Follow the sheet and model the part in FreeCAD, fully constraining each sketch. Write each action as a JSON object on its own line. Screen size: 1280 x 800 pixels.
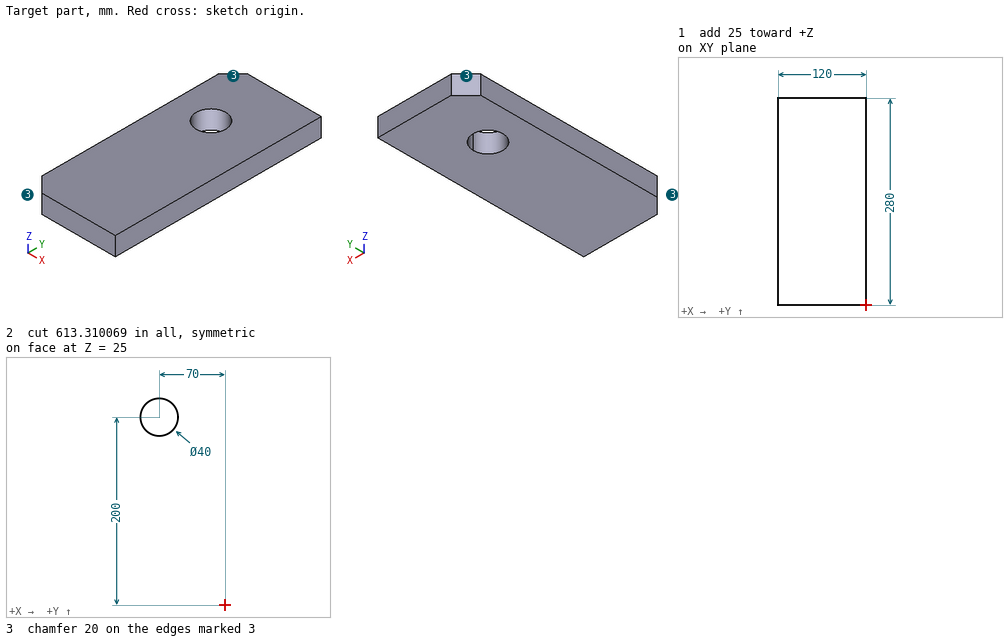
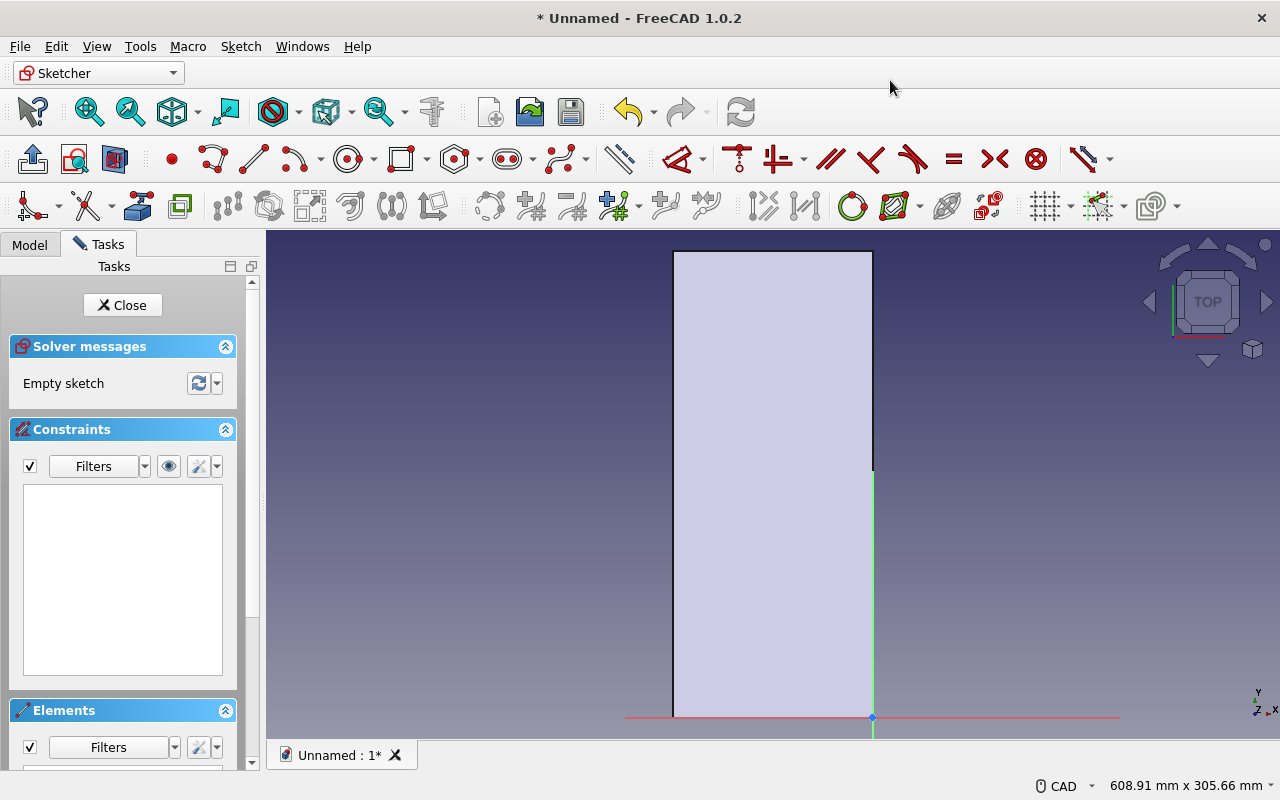
{"action": "scroll", "coordinate": [769, 359], "scroll_direction": "up", "scroll_amount": 8}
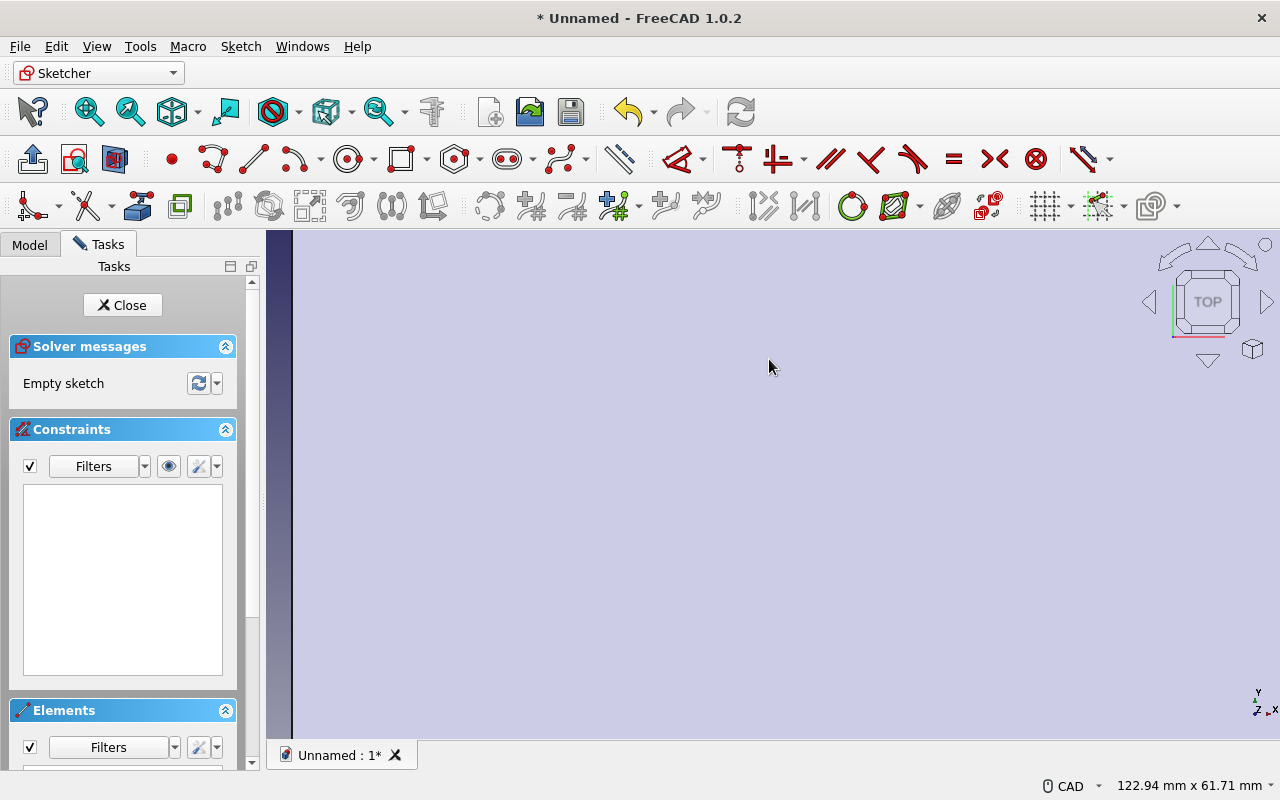
{"action": "left_click", "coordinate": [348, 160]}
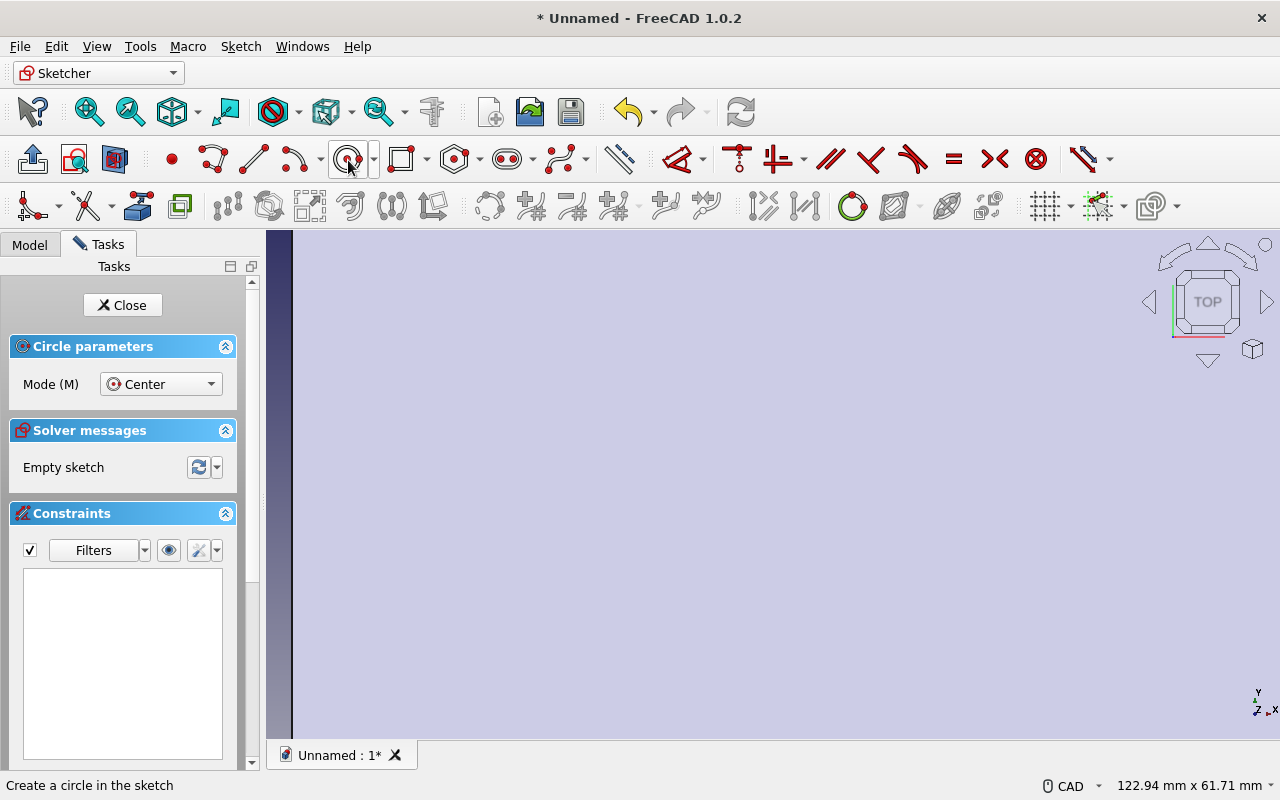
{"action": "left_click", "coordinate": [704, 485]}
{"action": "left_click", "coordinate": [821, 368]}
{"action": "key", "text": "Escape"}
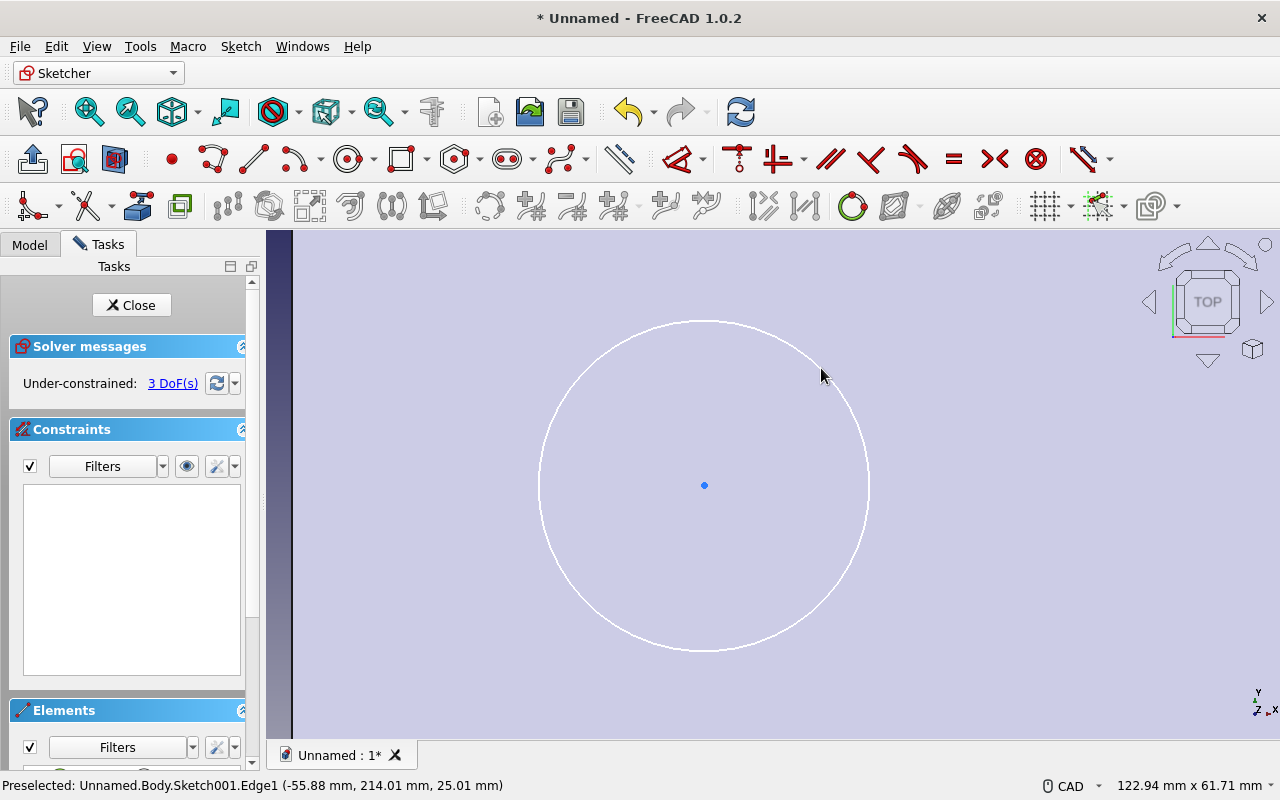
{"action": "left_click", "coordinate": [821, 369]}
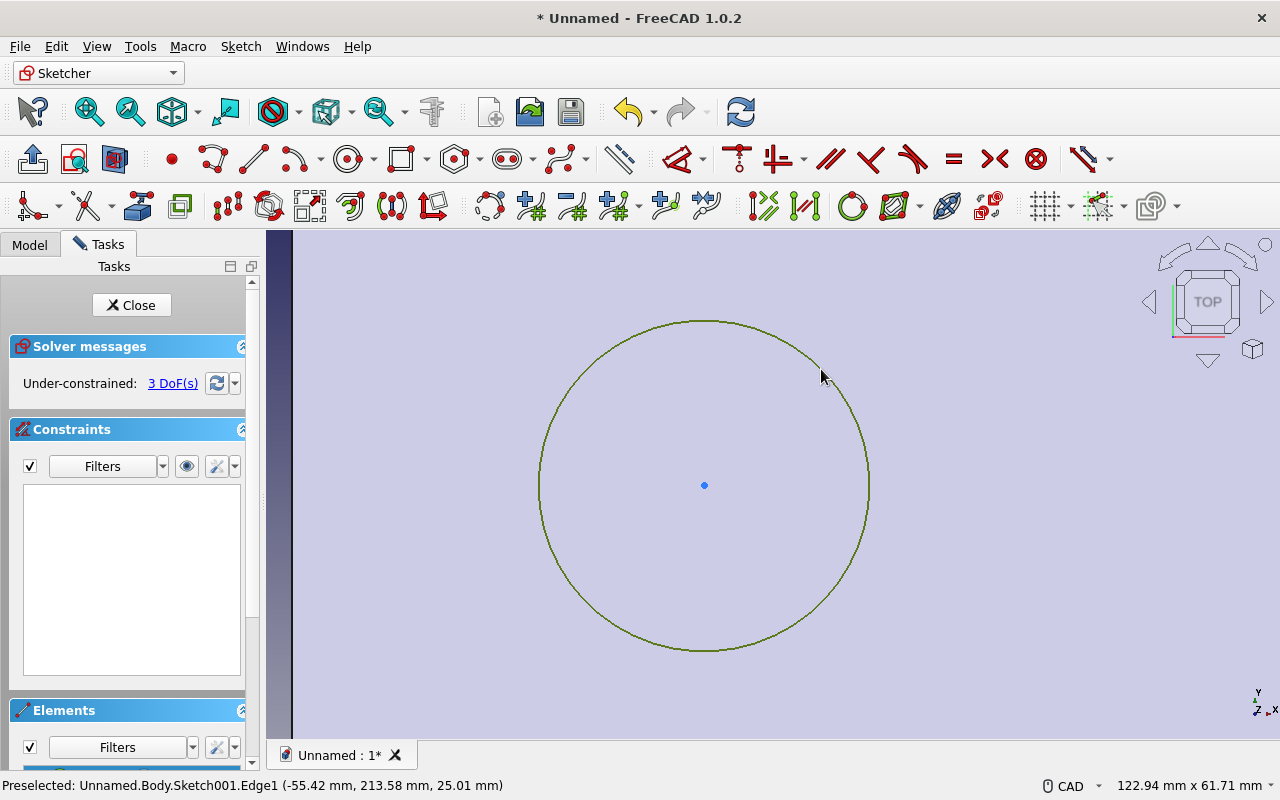
{"action": "left_click", "coordinate": [702, 160]}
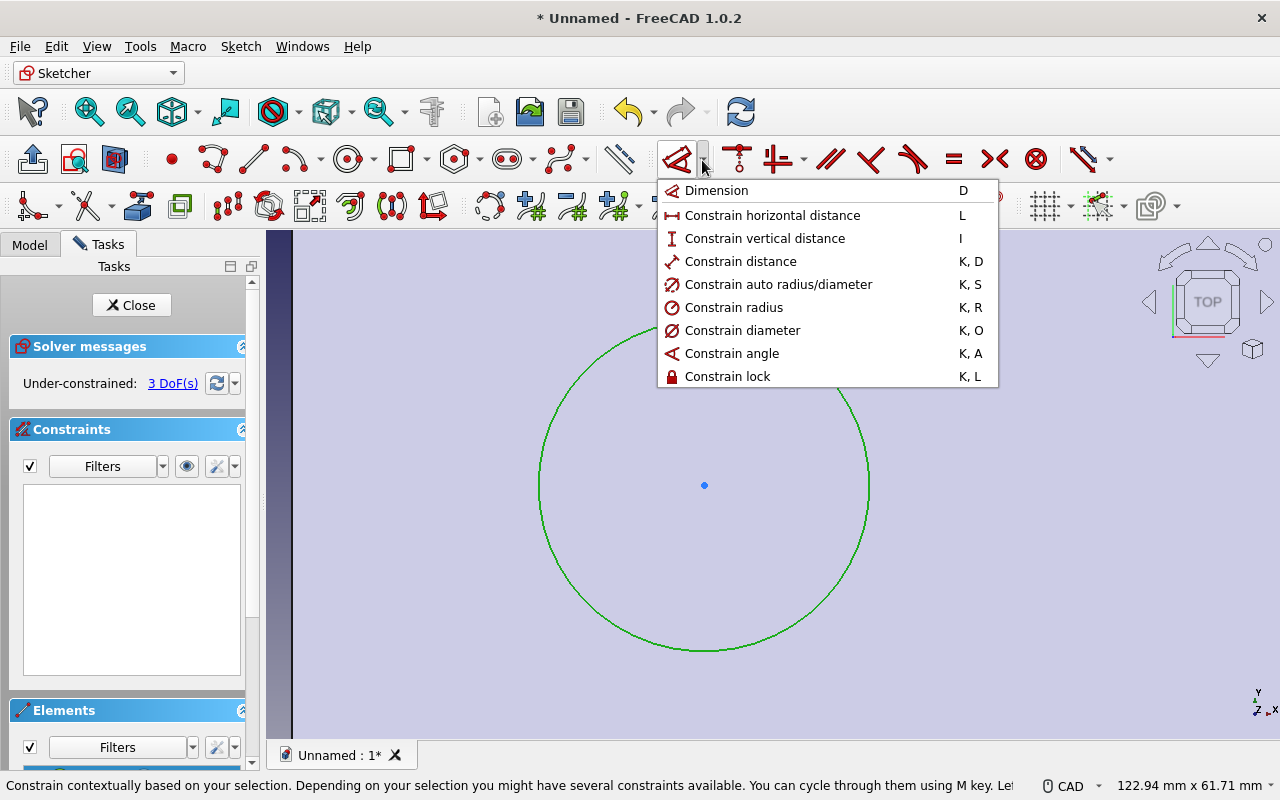
{"action": "left_click", "coordinate": [828, 330]}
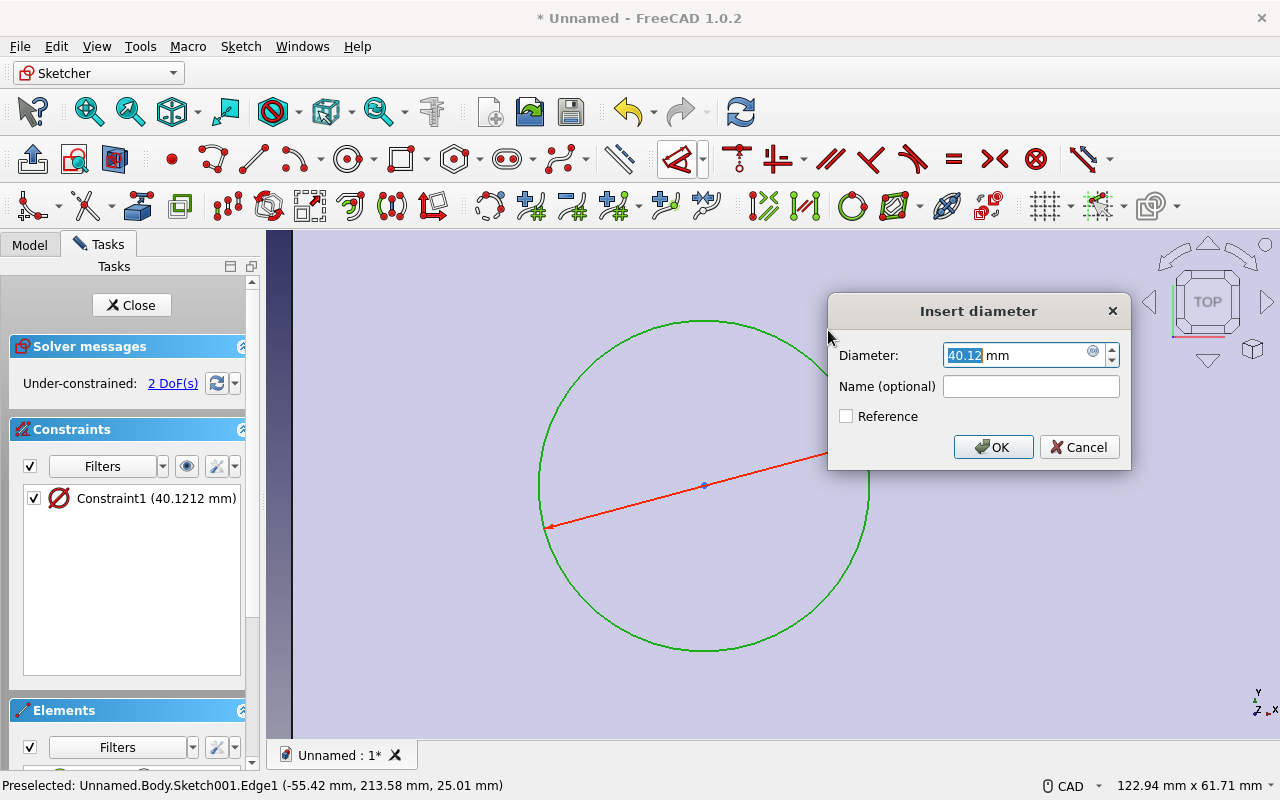
{"action": "type", "text": "40"}
{"action": "key", "text": "Return"}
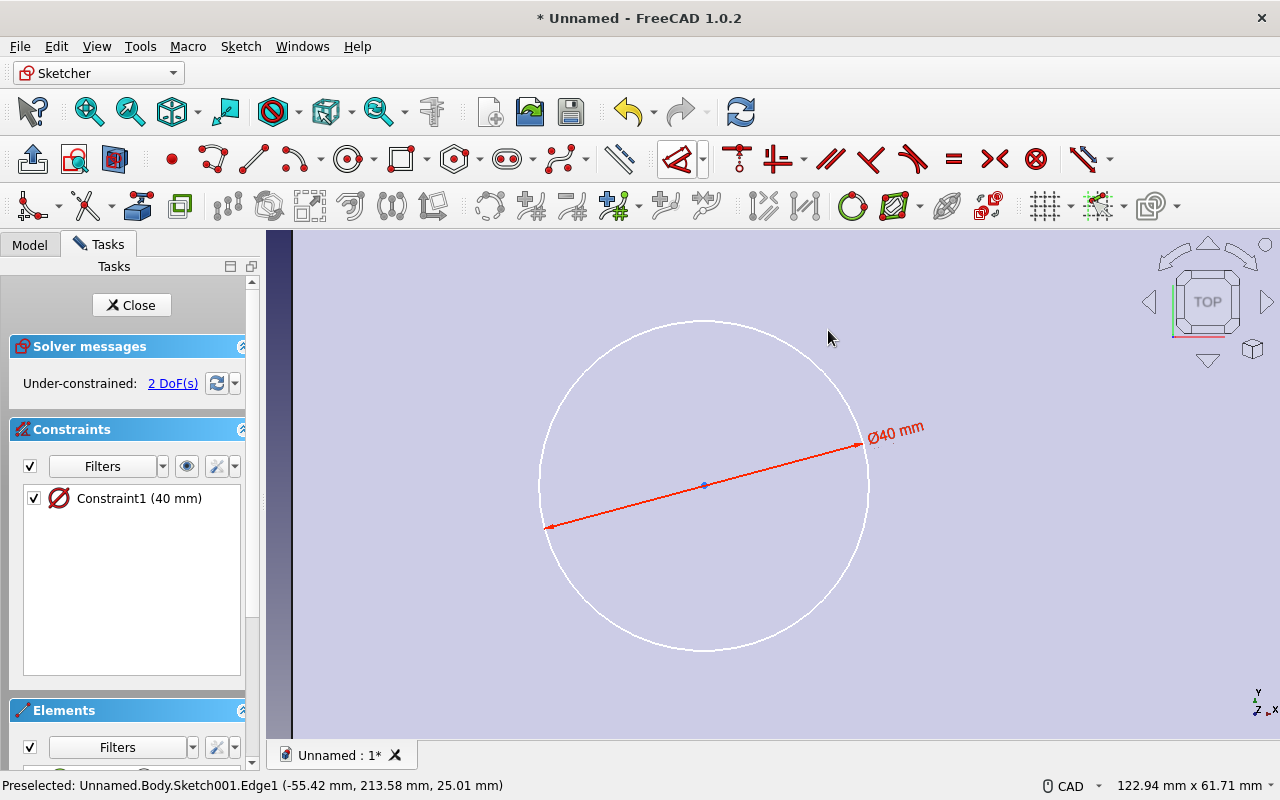
{"action": "left_click", "coordinate": [704, 486]}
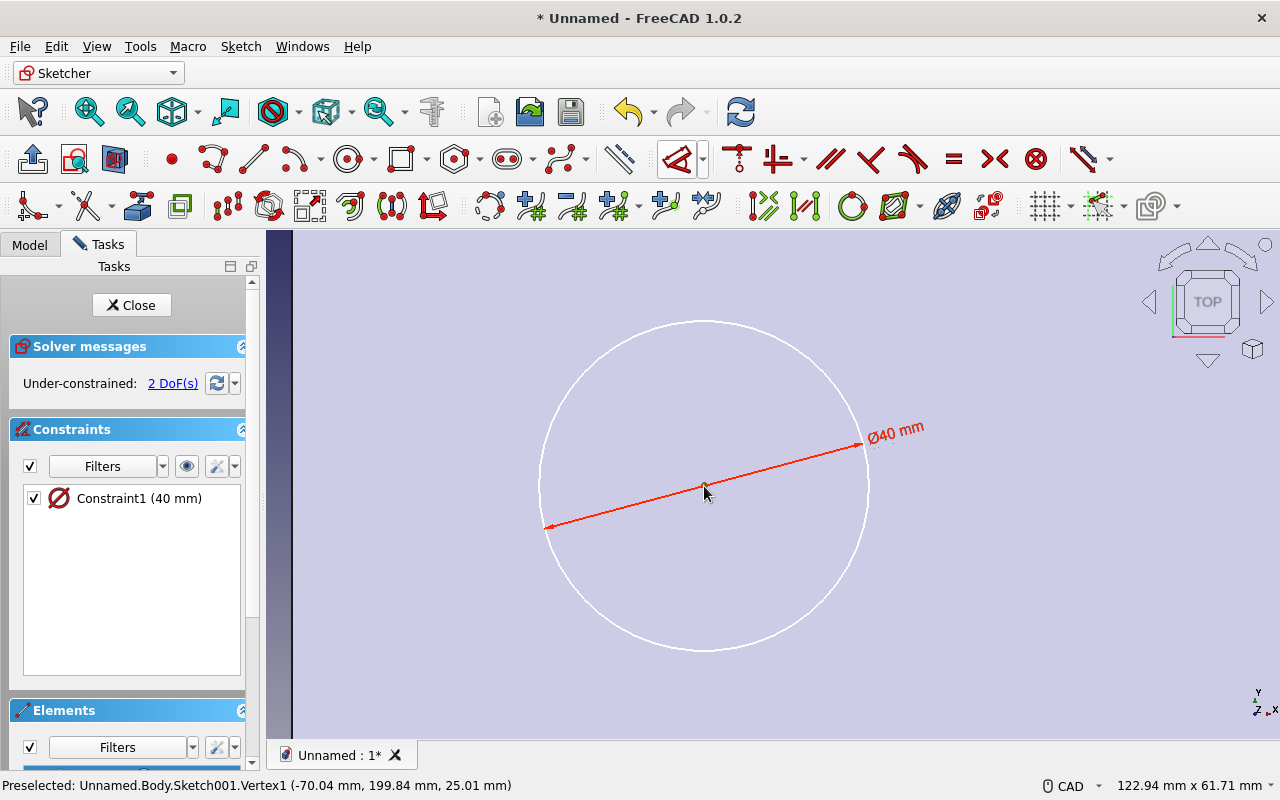
{"action": "left_click", "coordinate": [702, 160]}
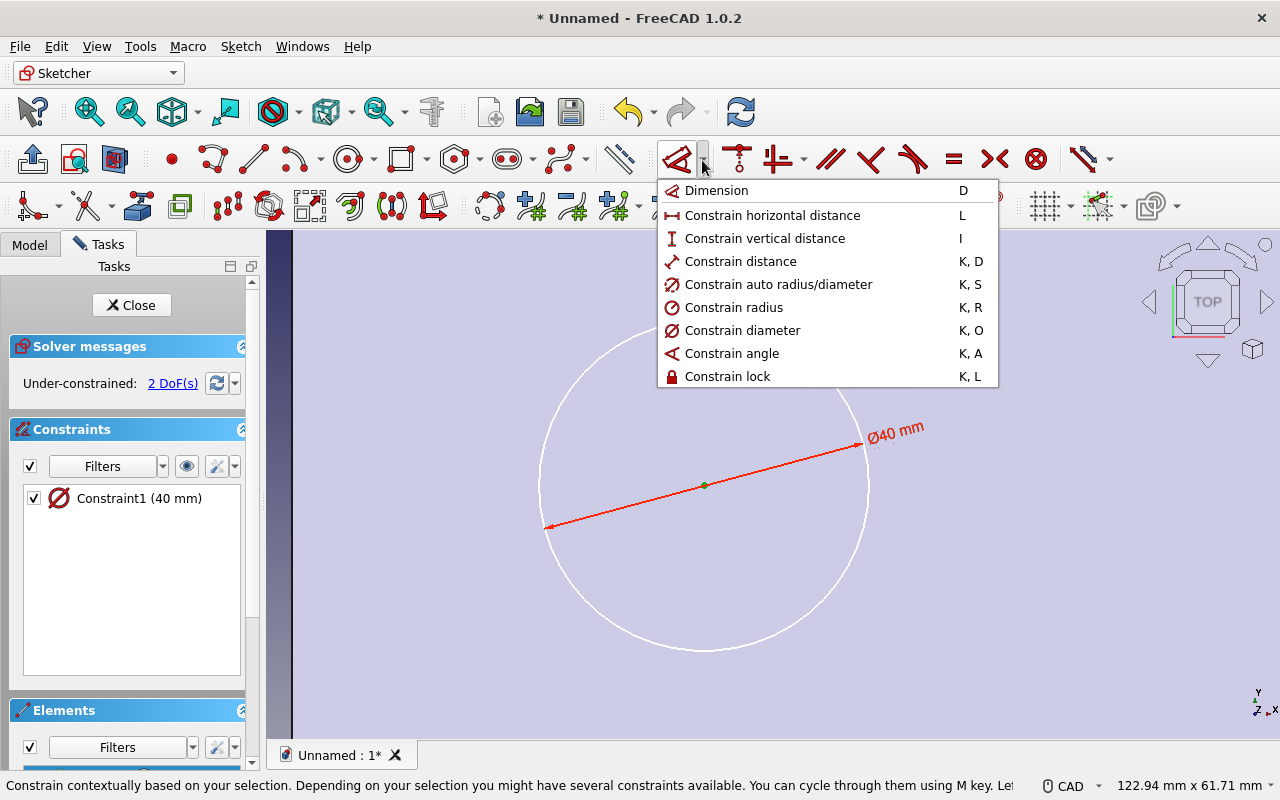
{"action": "left_click", "coordinate": [828, 216]}